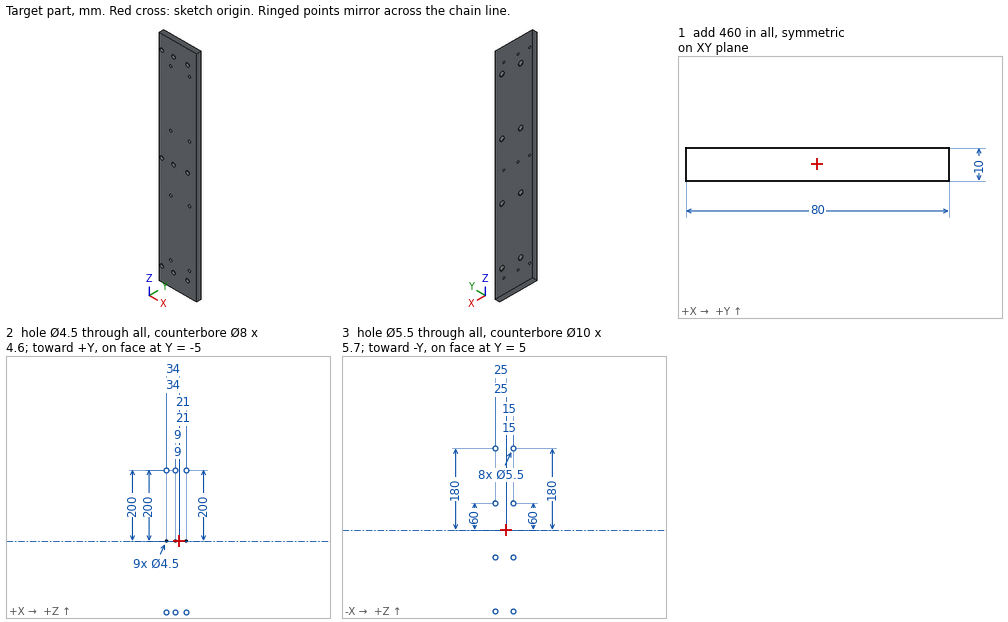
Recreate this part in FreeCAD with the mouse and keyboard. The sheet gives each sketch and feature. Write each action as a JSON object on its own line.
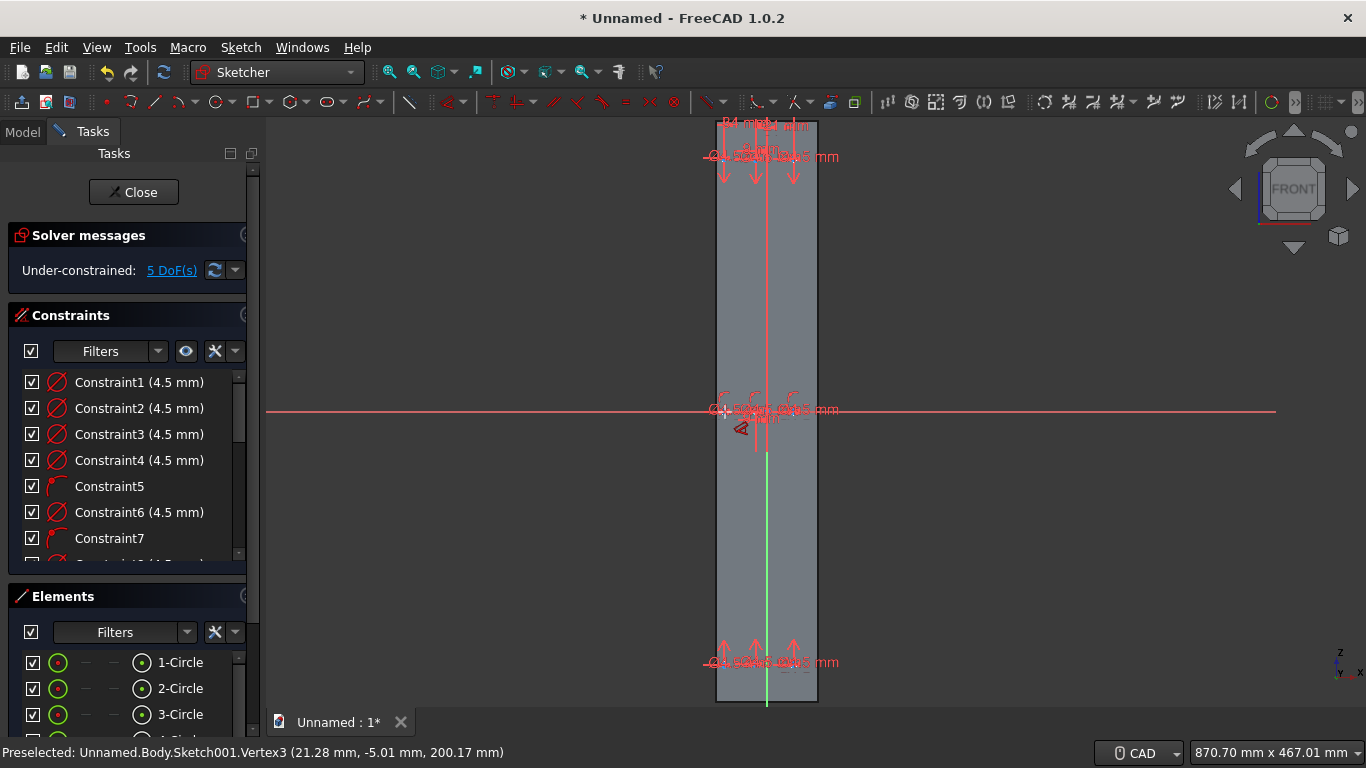
{"action": "left_click", "coordinate": [724, 412]}
{"action": "left_click", "coordinate": [746, 446]}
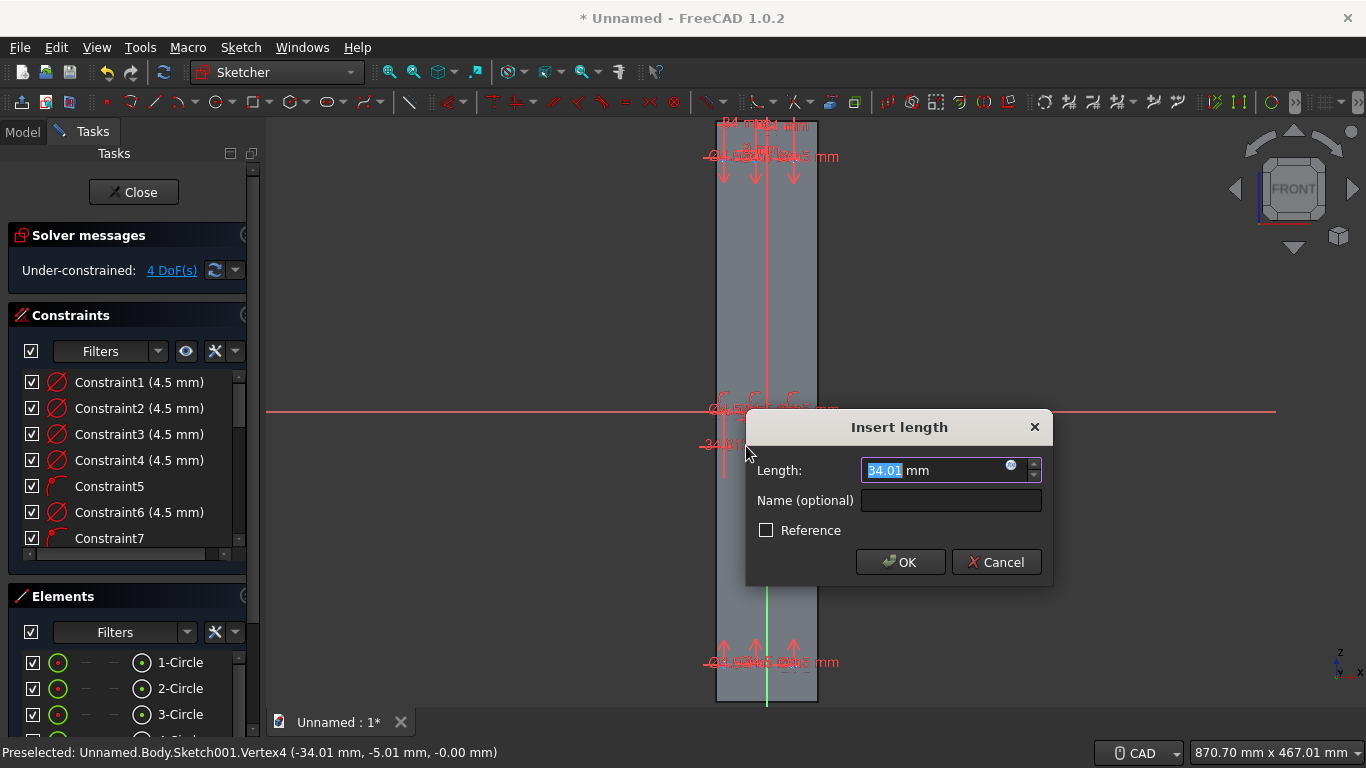
{"action": "type", "text": "34"}
{"action": "key", "text": "Return"}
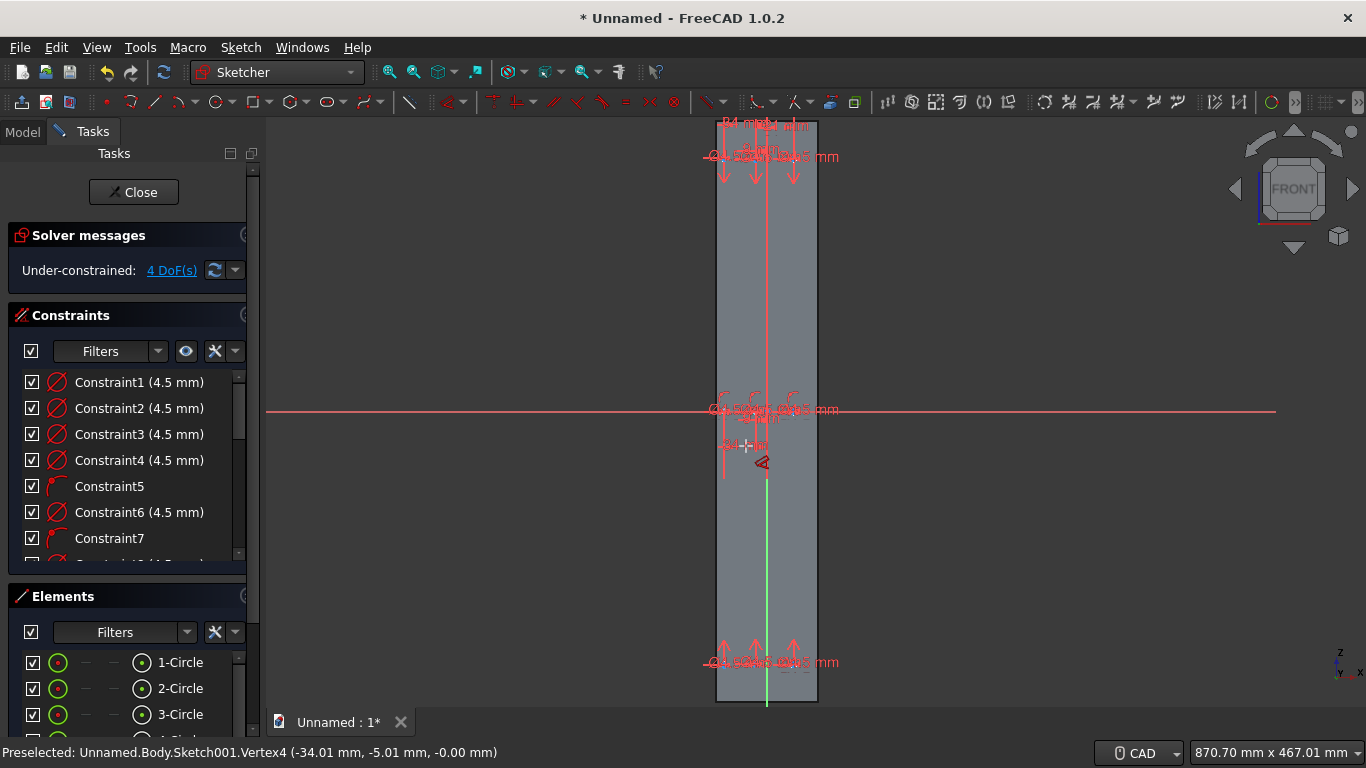
{"action": "scroll", "coordinate": [794, 412], "scroll_direction": "up", "scroll_amount": 3}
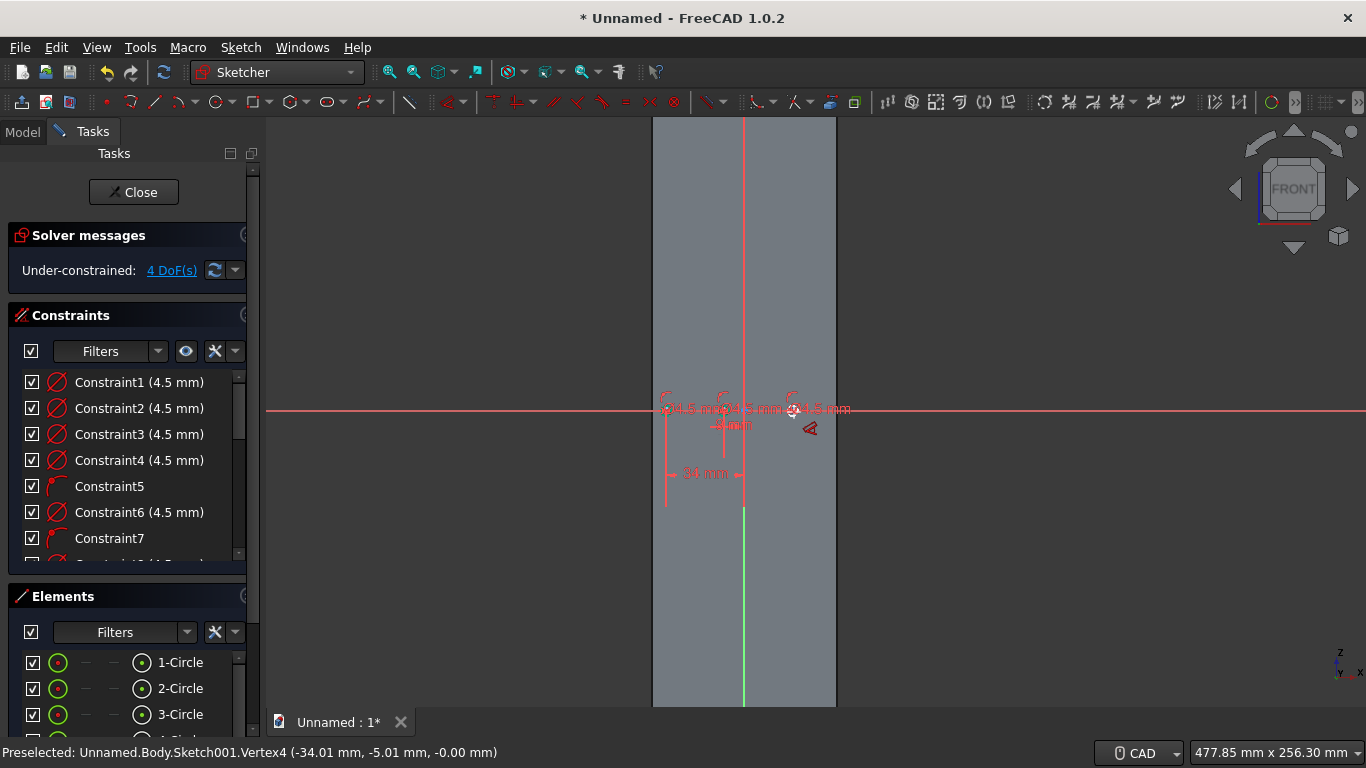
{"action": "left_click", "coordinate": [793, 411]}
{"action": "left_click", "coordinate": [769, 377]}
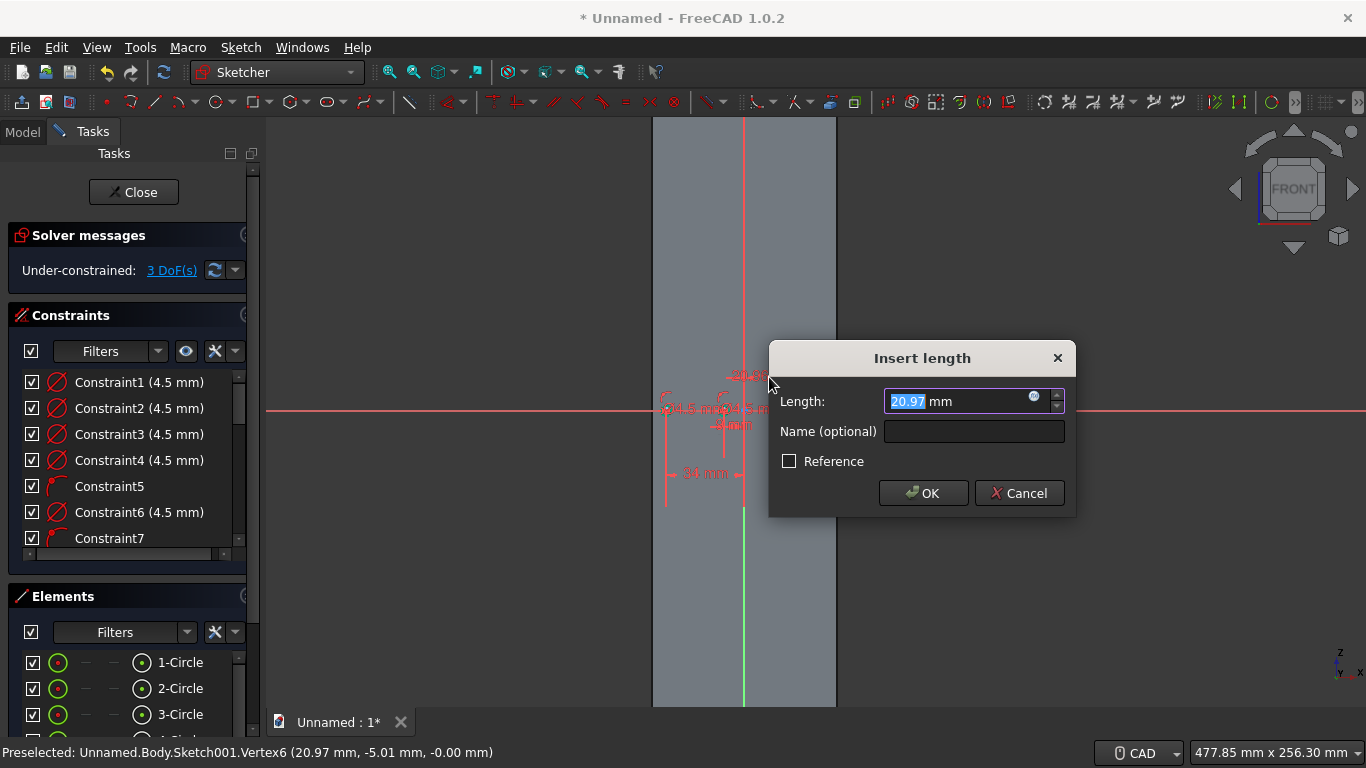
{"action": "type", "text": "21"}
{"action": "key", "text": "Return"}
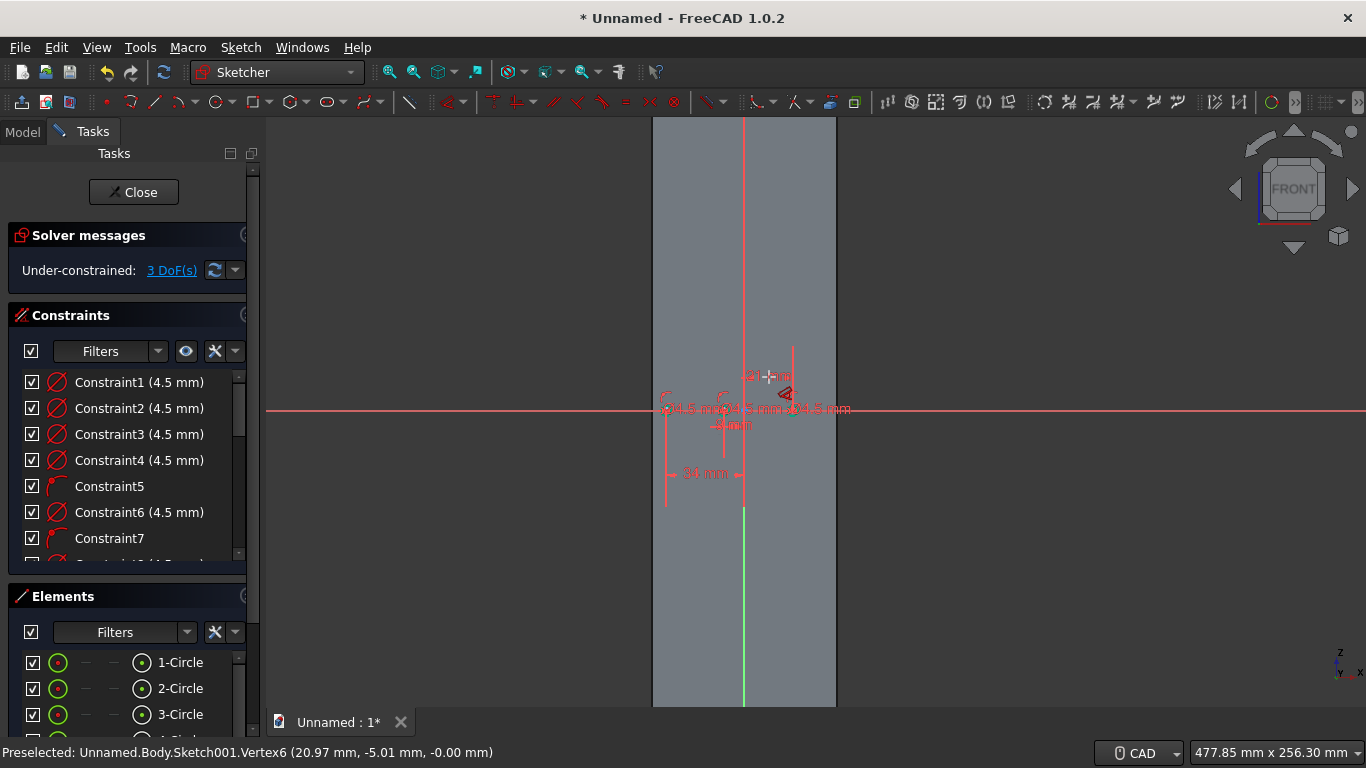
{"action": "scroll", "coordinate": [758, 413], "scroll_direction": "down", "scroll_amount": 5}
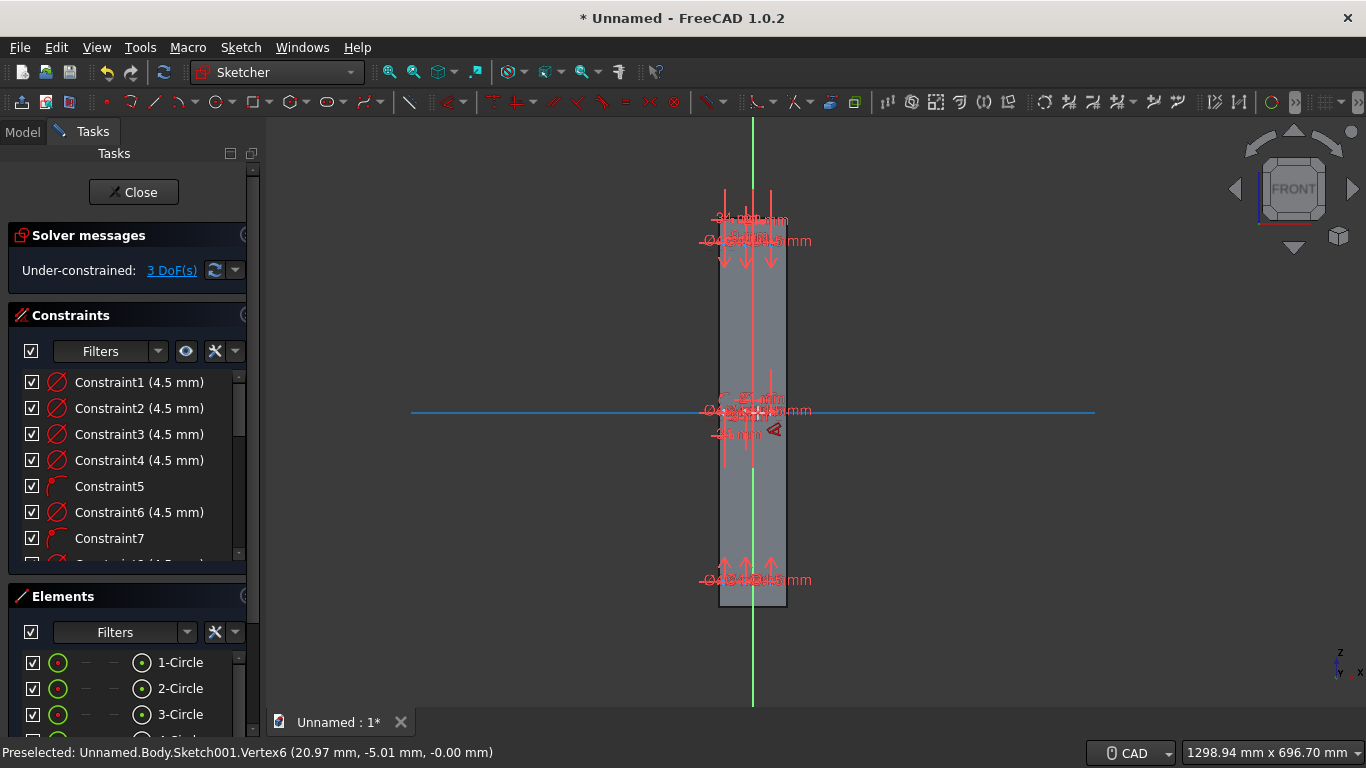
{"action": "left_click", "coordinate": [725, 243]}
{"action": "left_click", "coordinate": [691, 328]}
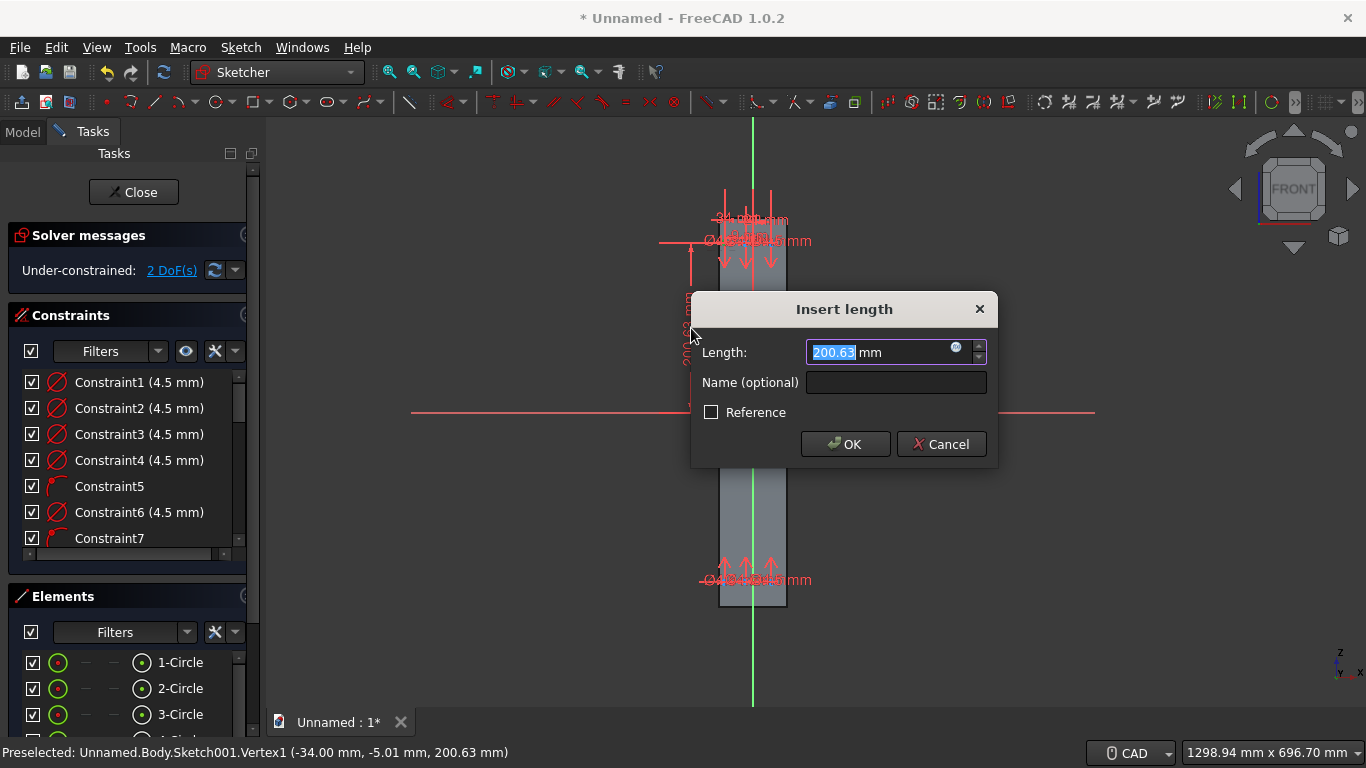
{"action": "type", "text": "200"}
{"action": "key", "text": "Return"}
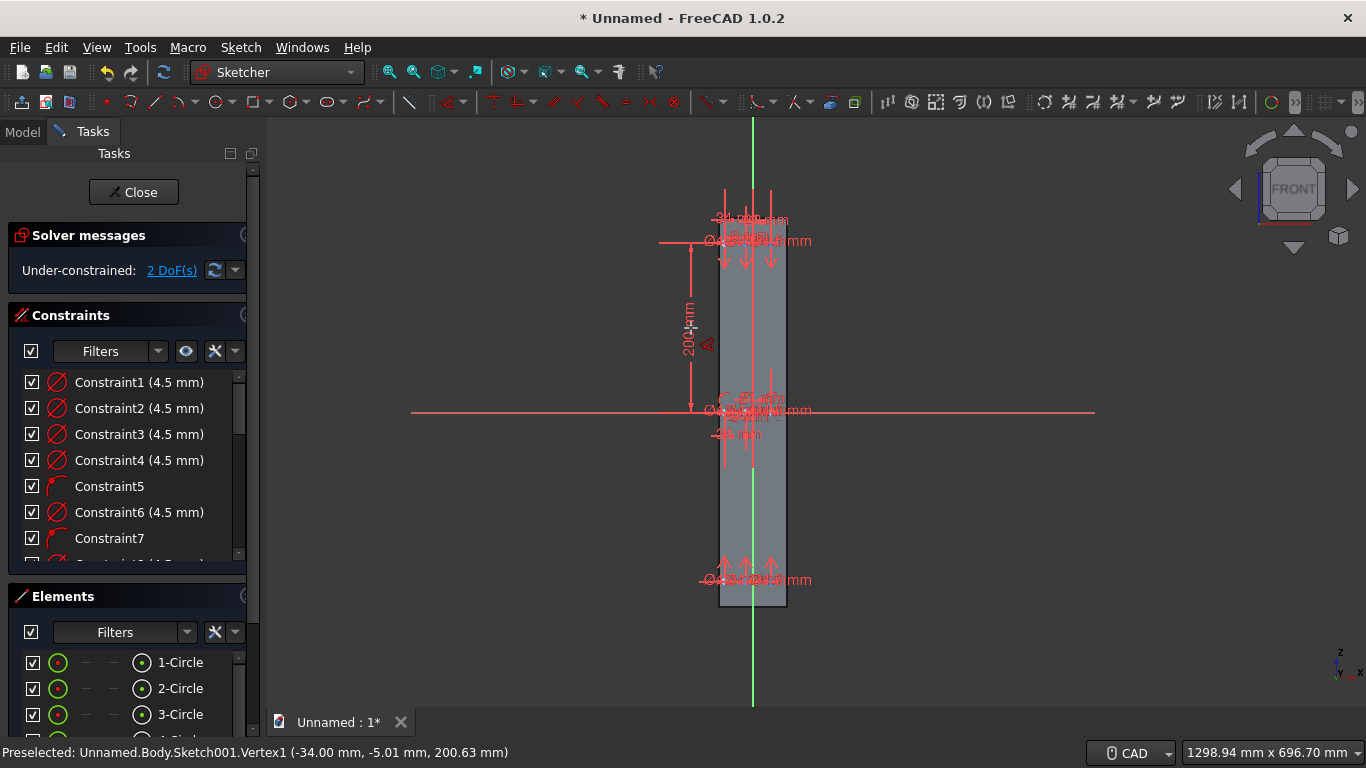
{"action": "left_click", "coordinate": [746, 243]}
{"action": "left_click", "coordinate": [787, 328]}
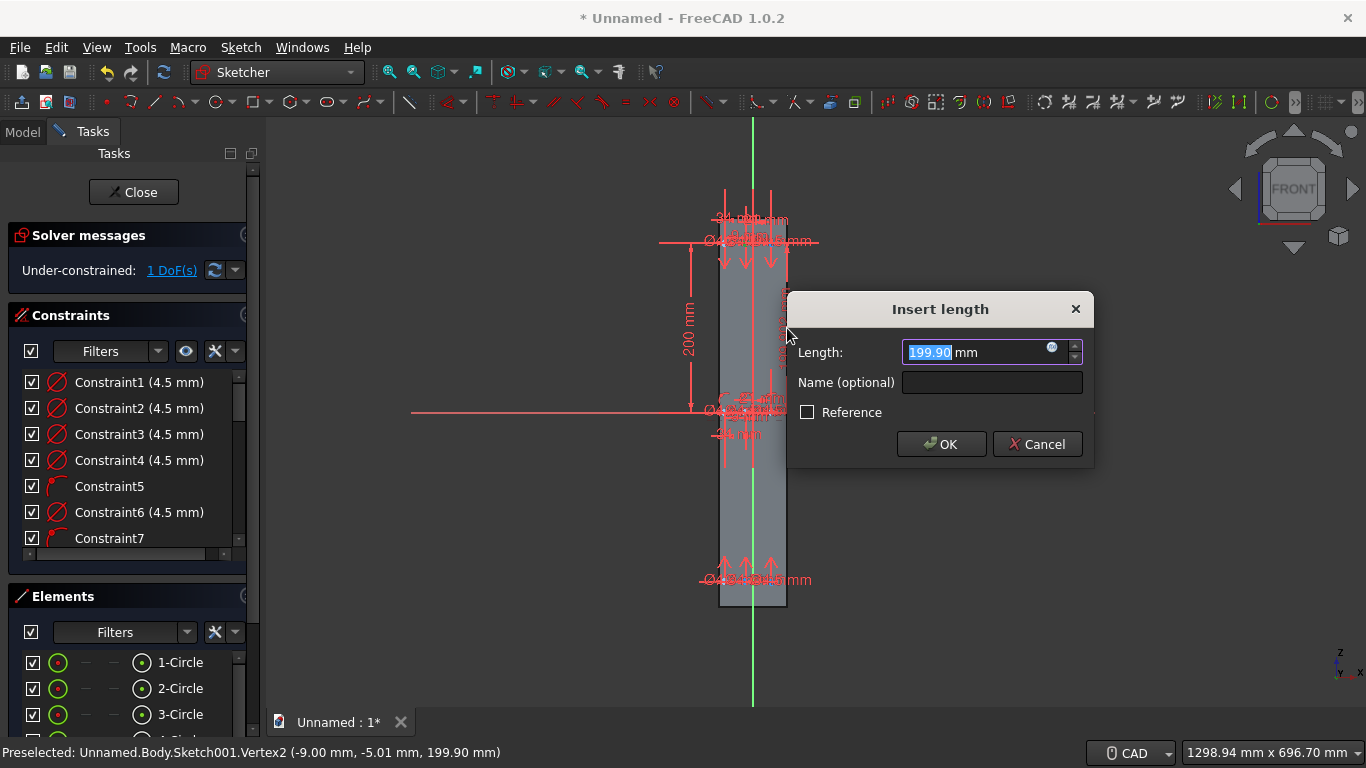
{"action": "type", "text": "200"}
{"action": "key", "text": "Return"}